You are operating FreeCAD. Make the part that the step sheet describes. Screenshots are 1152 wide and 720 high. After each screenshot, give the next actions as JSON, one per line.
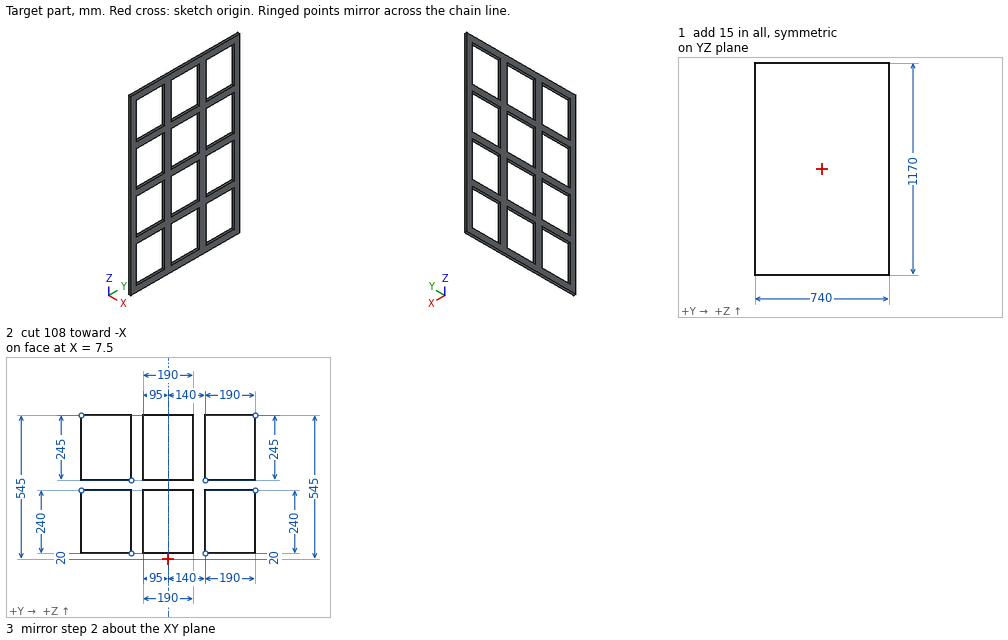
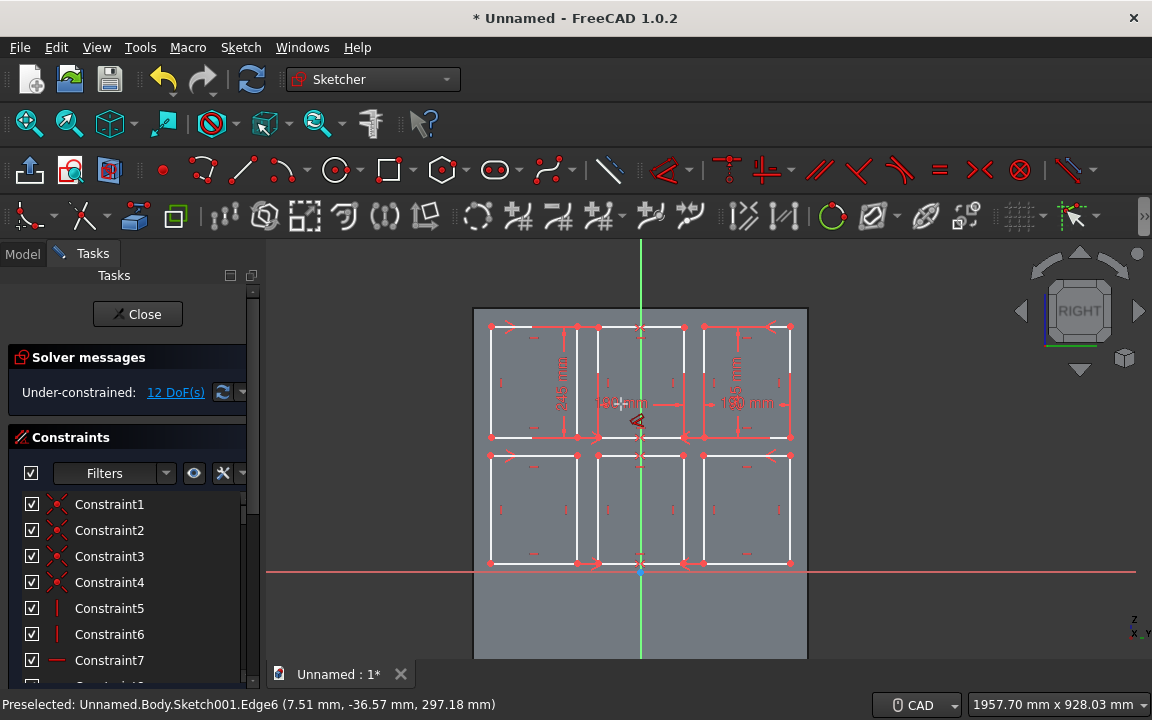
{"action": "left_click", "coordinate": [598, 488]}
{"action": "left_click", "coordinate": [564, 510]}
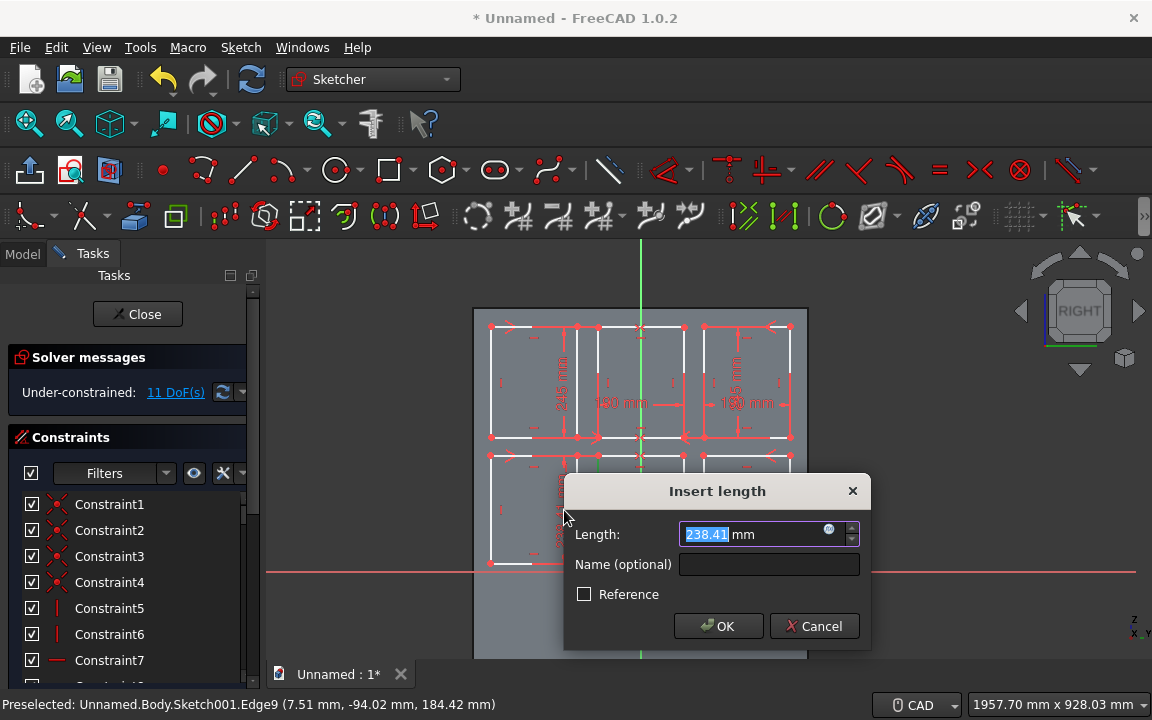
{"action": "type", "text": "240"}
{"action": "key", "text": "Return"}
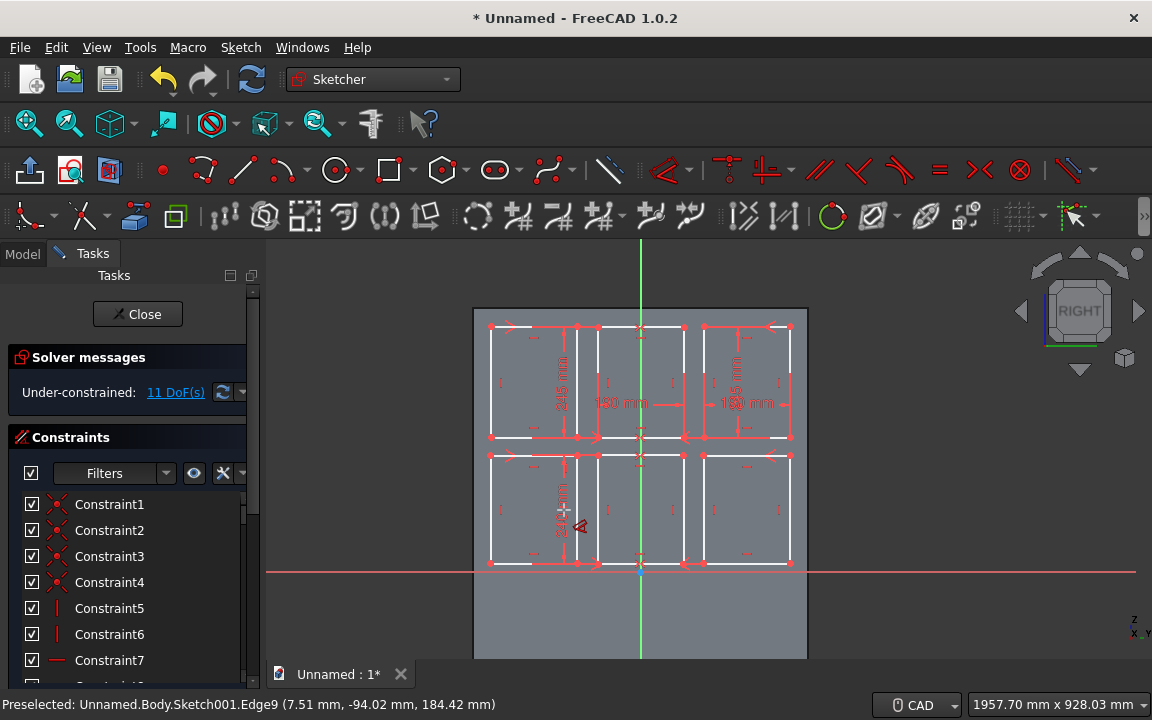
{"action": "scroll", "coordinate": [624, 564], "scroll_direction": "up", "scroll_amount": 3}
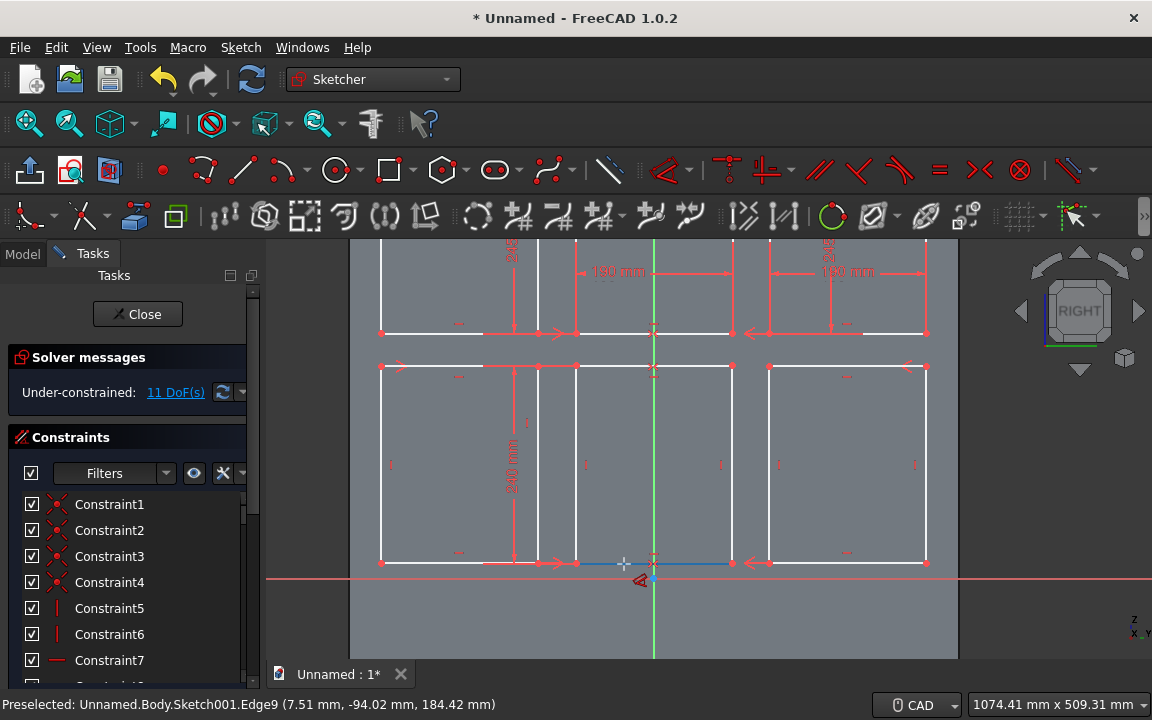
{"action": "left_click", "coordinate": [623, 564]}
{"action": "left_click", "coordinate": [618, 598]}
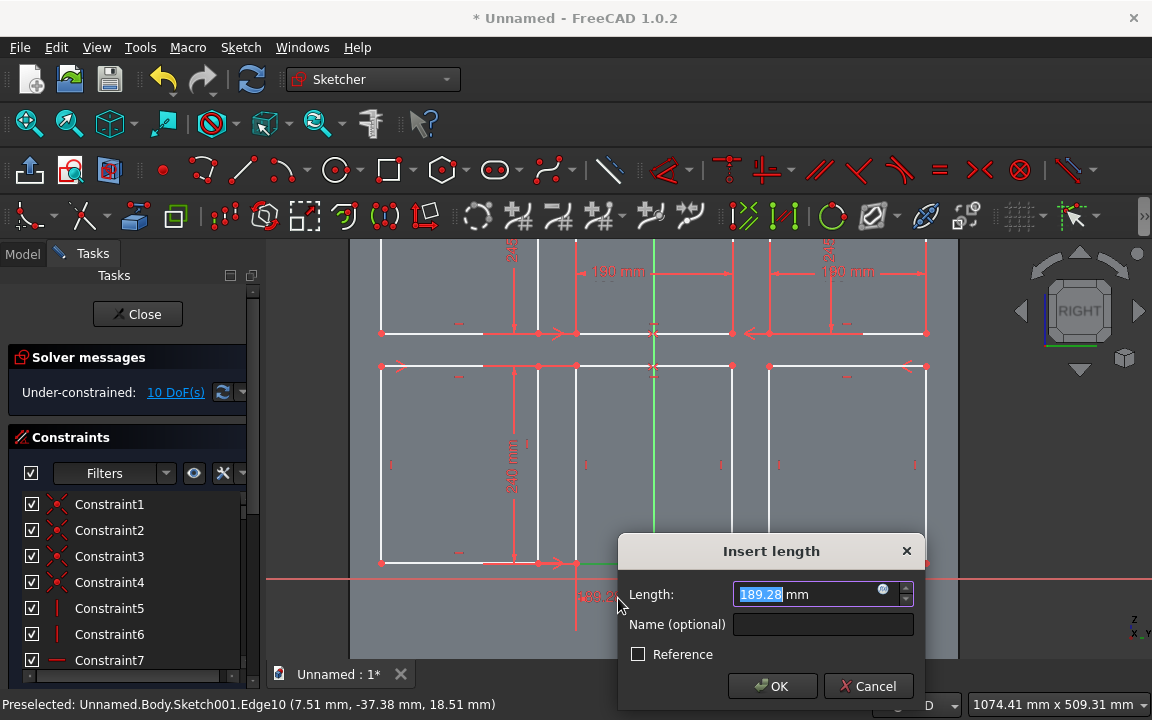
{"action": "type", "text": "190"}
{"action": "key", "text": "Return"}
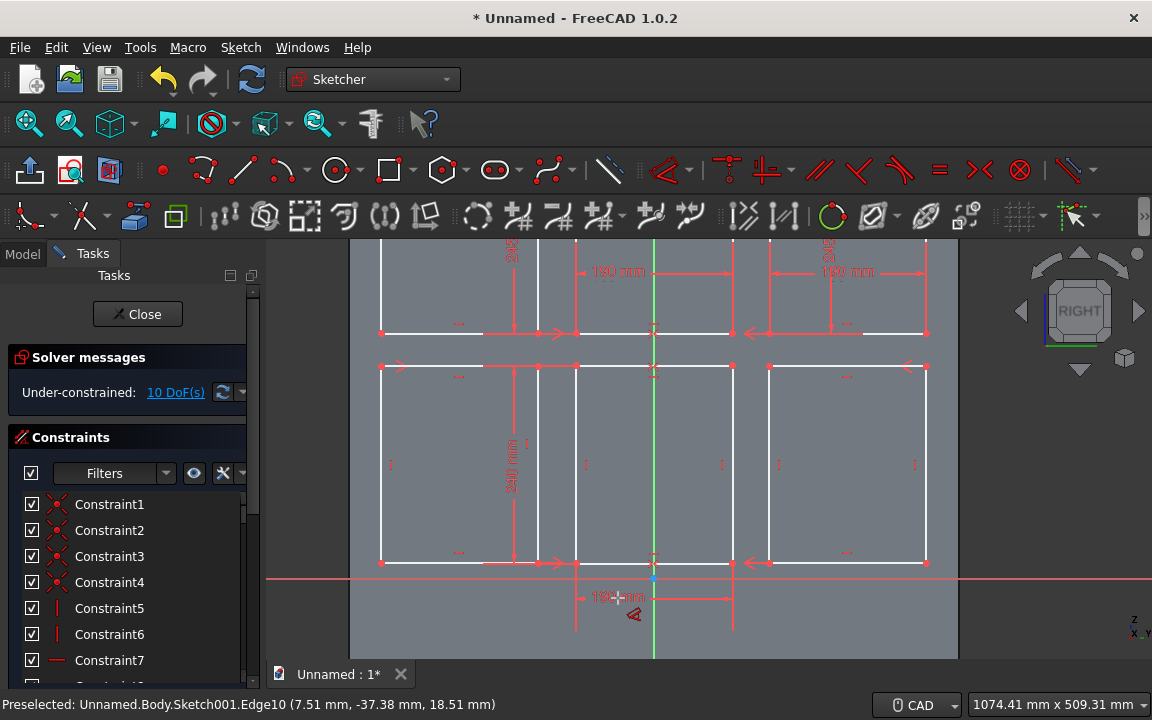
{"action": "left_click", "coordinate": [769, 425]}
{"action": "left_click", "coordinate": [803, 465]}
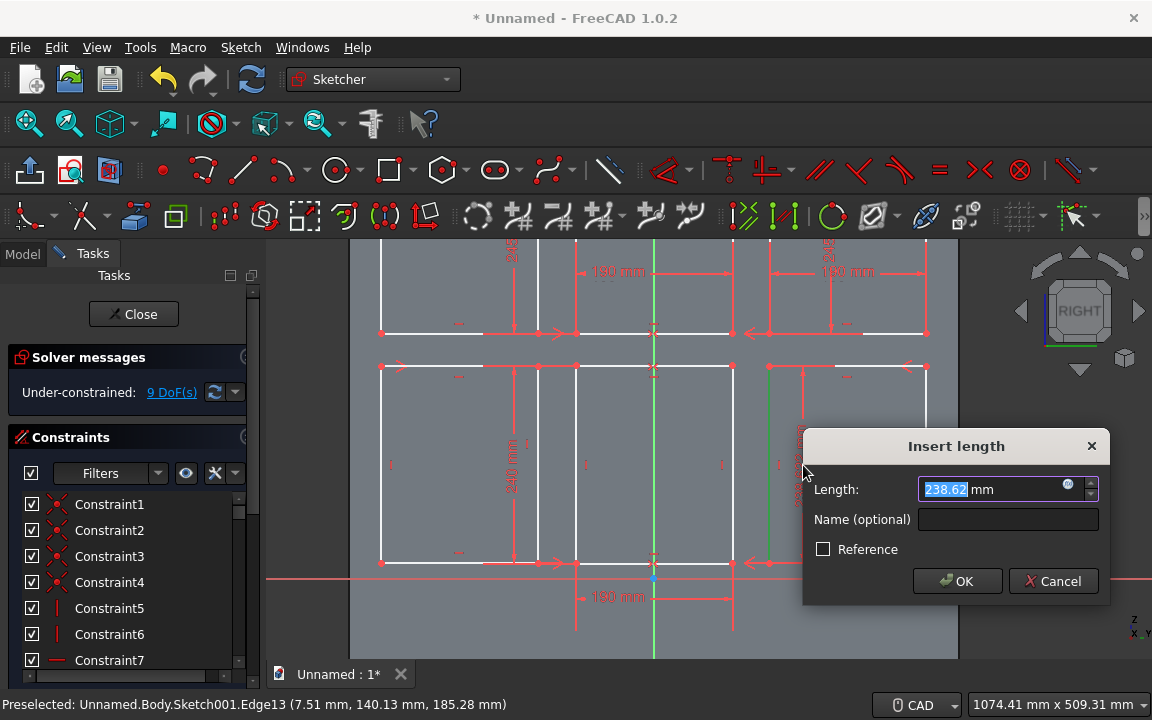
{"action": "type", "text": "240"}
{"action": "key", "text": "Return"}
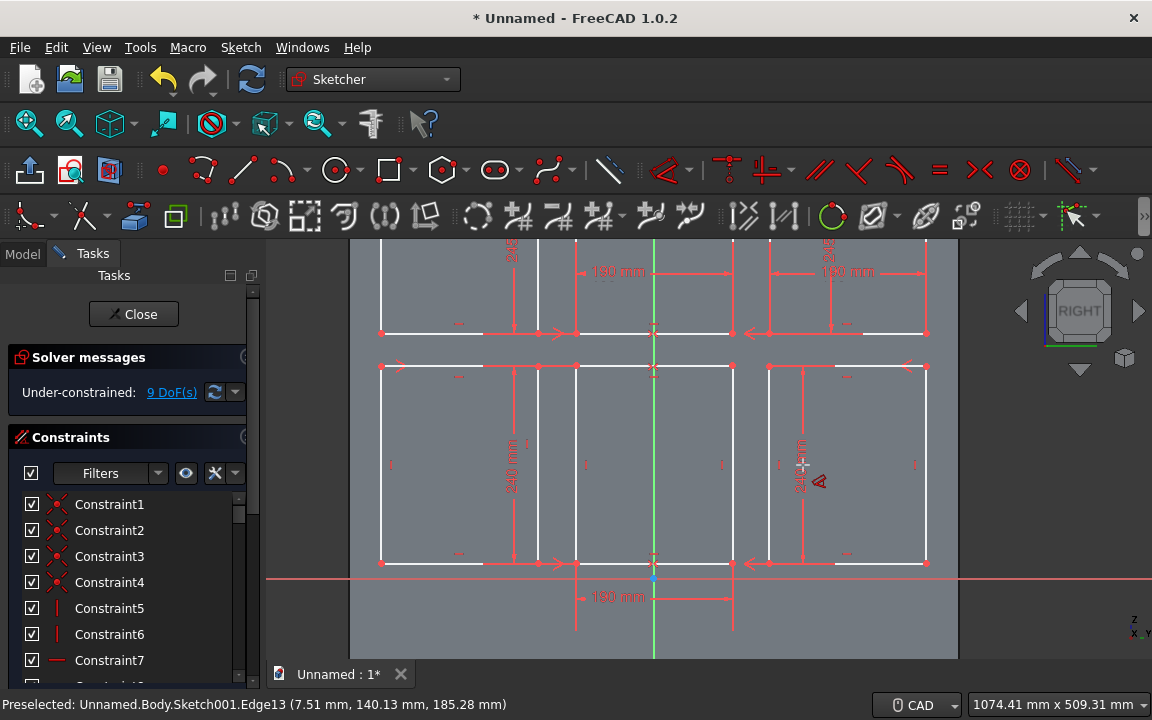
{"action": "left_click", "coordinate": [816, 564]}
{"action": "left_click", "coordinate": [848, 598]}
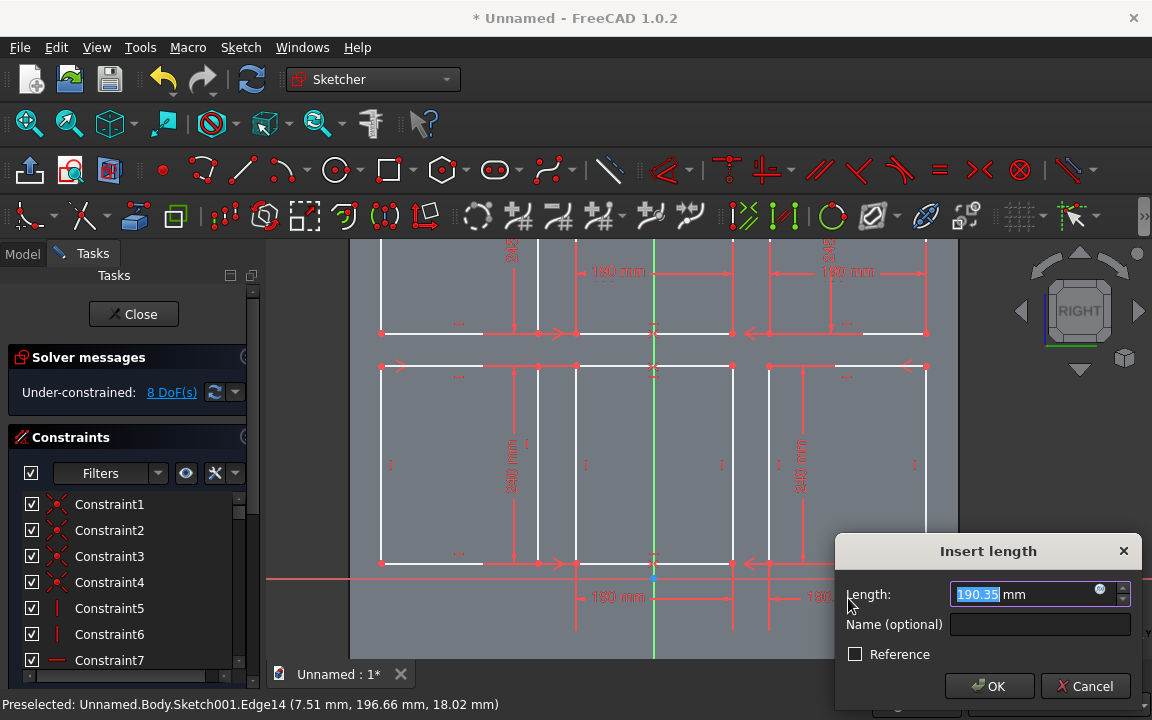
{"action": "type", "text": "190"}
{"action": "key", "text": "Return"}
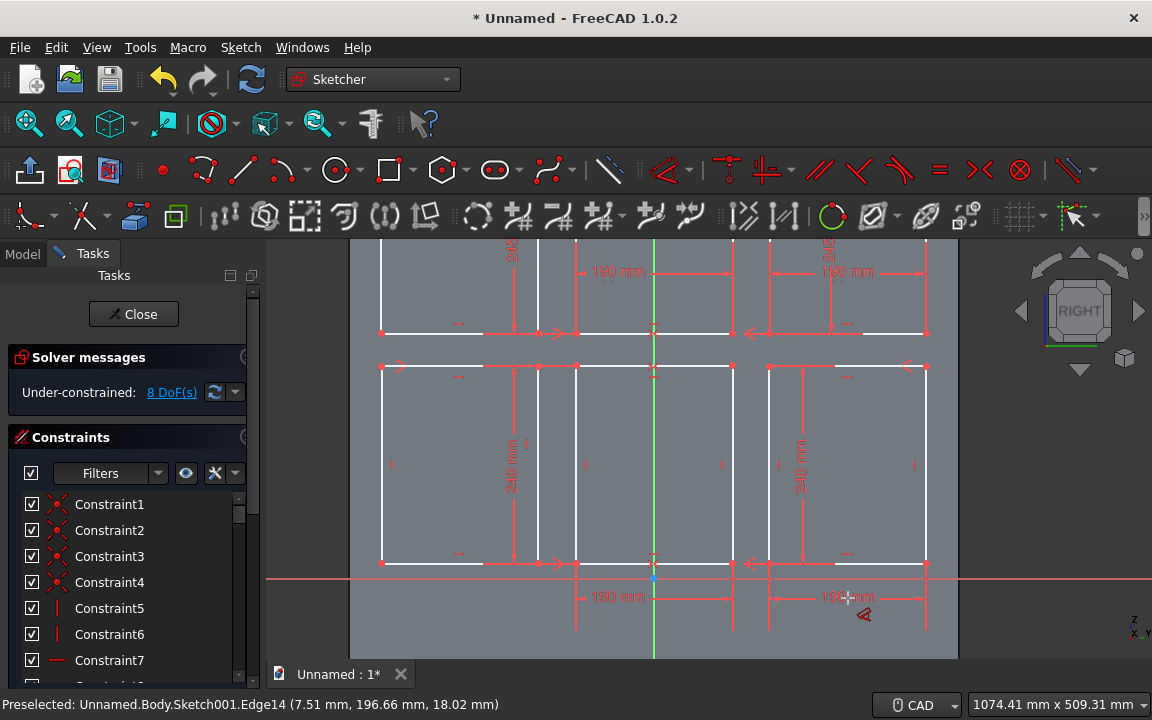
{"action": "scroll", "coordinate": [624, 564], "scroll_direction": "down", "scroll_amount": 3}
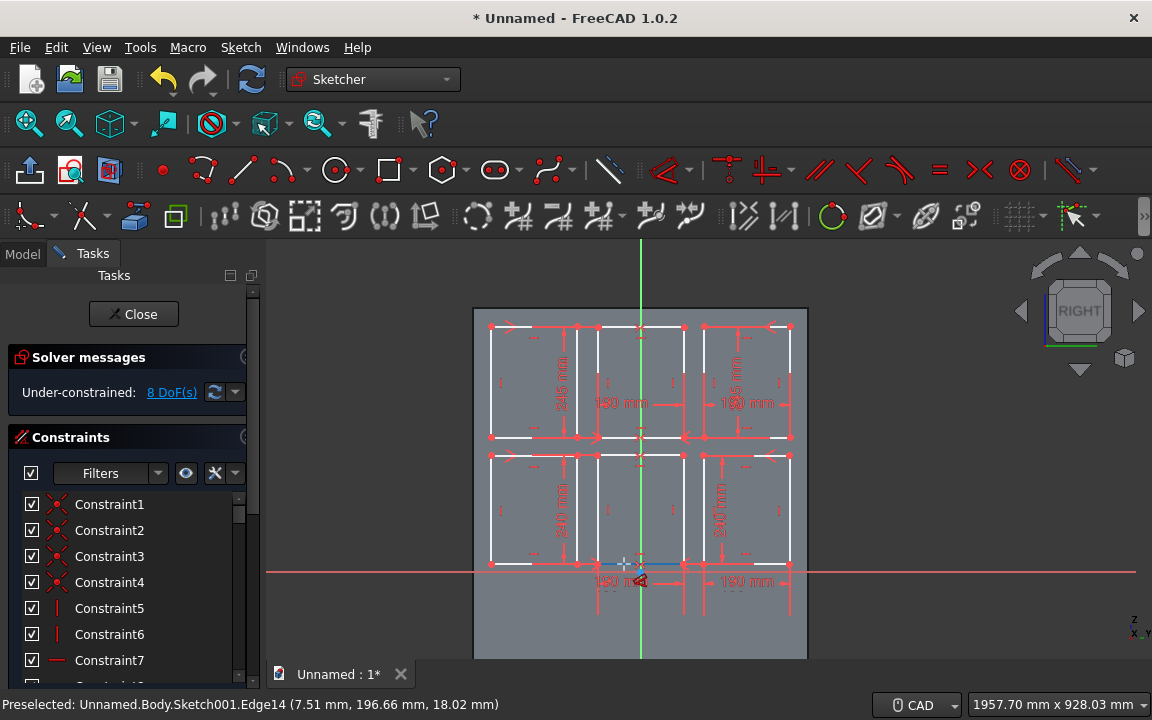
{"action": "left_click", "coordinate": [598, 327]}
{"action": "left_click", "coordinate": [619, 606]}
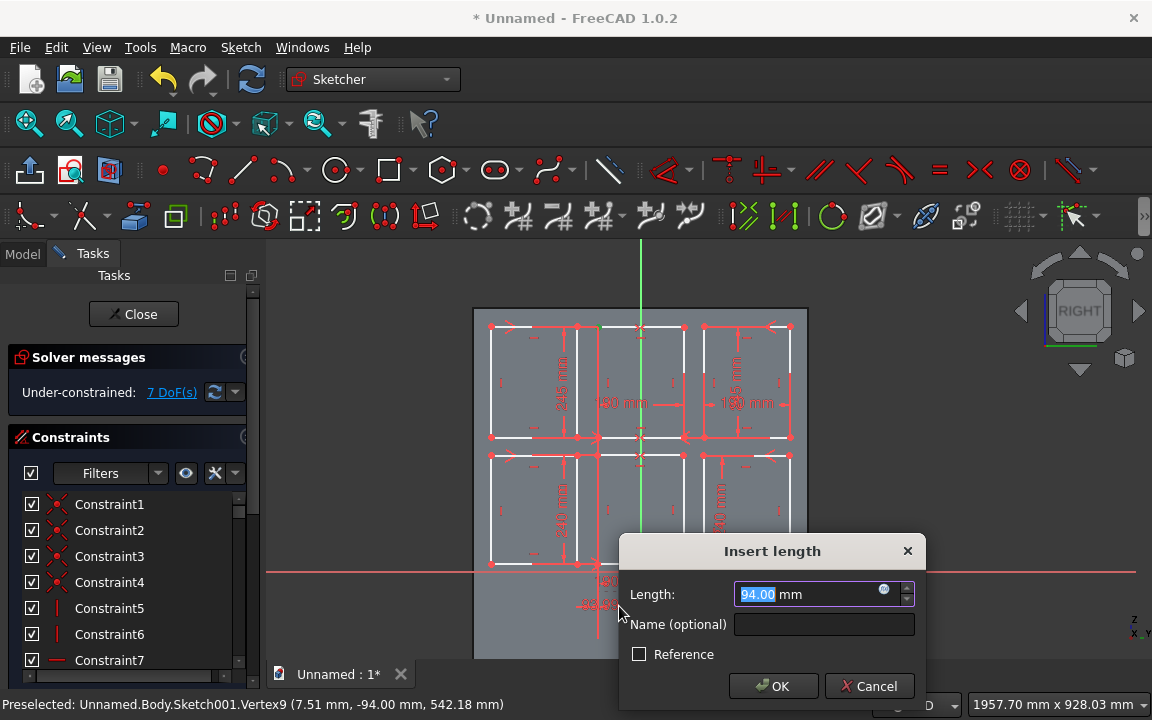
{"action": "type", "text": "95"}
{"action": "key", "text": "Return"}